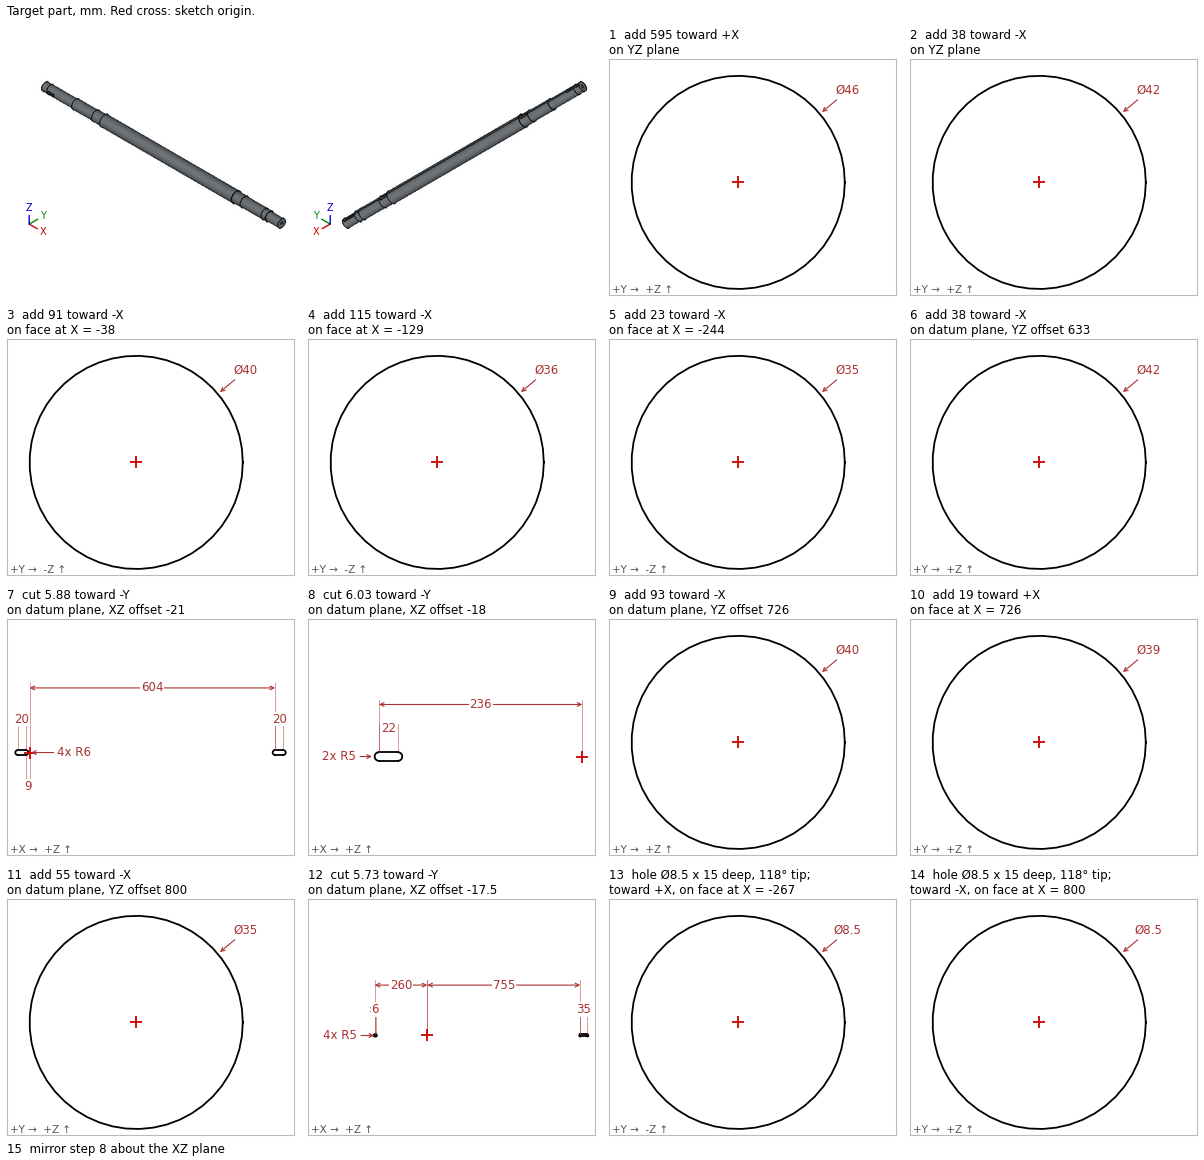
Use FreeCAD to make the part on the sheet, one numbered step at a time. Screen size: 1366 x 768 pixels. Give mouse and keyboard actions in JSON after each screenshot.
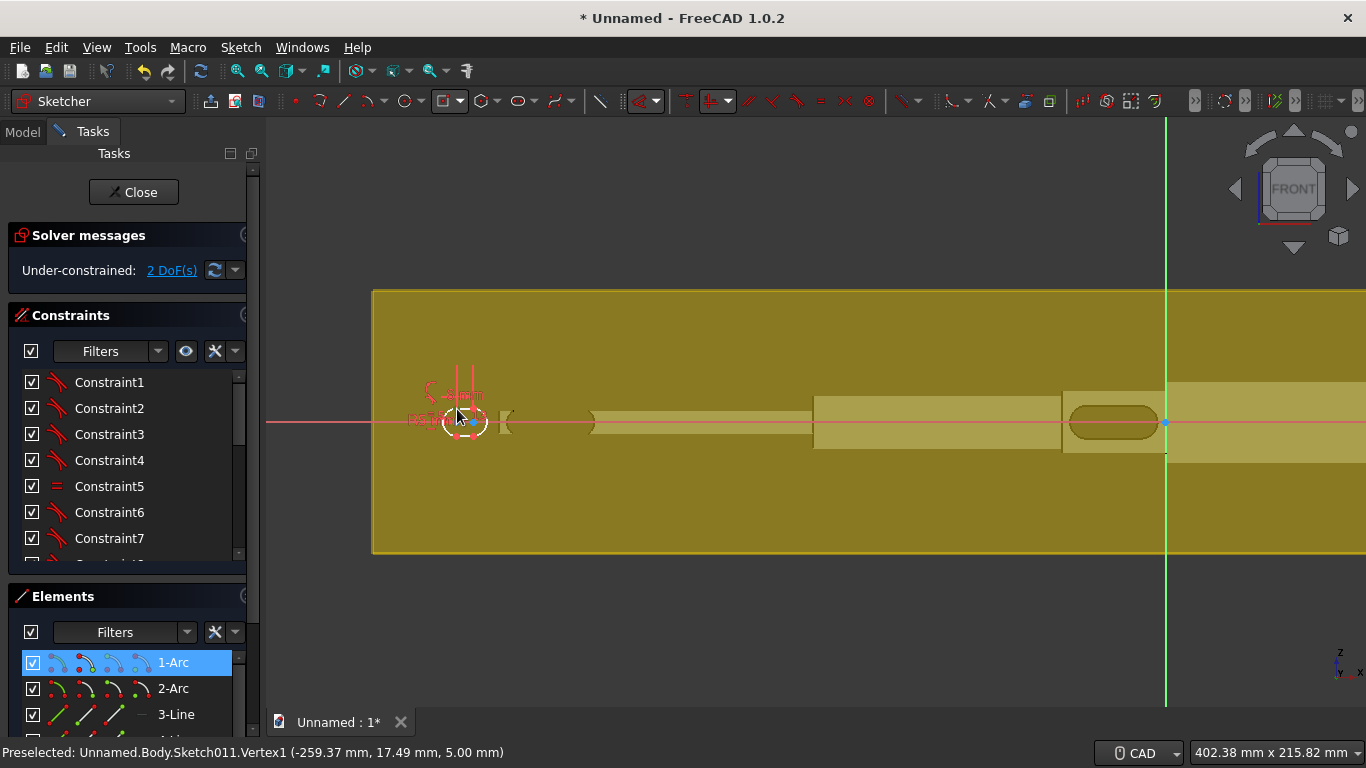
{"action": "key", "text": "l"}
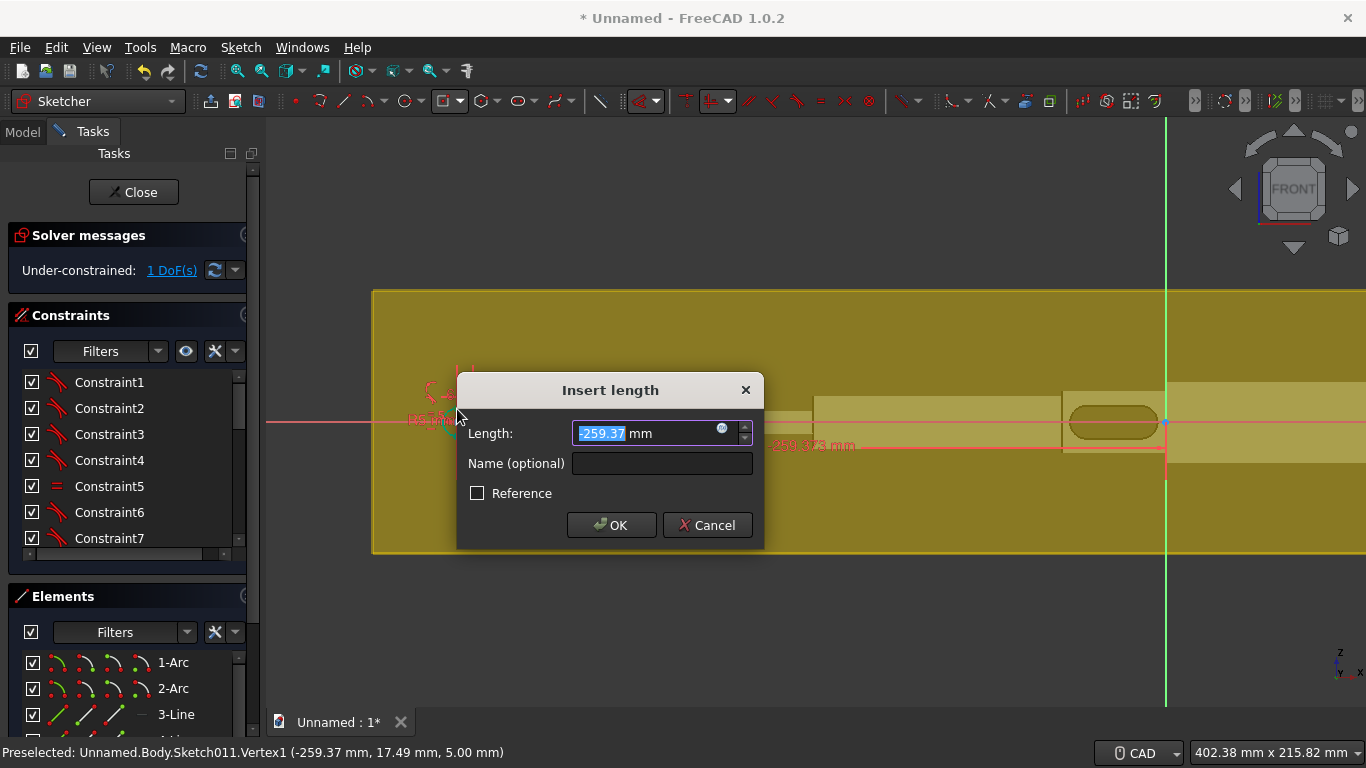
{"action": "type", "text": "-260"}
{"action": "key", "text": "Return"}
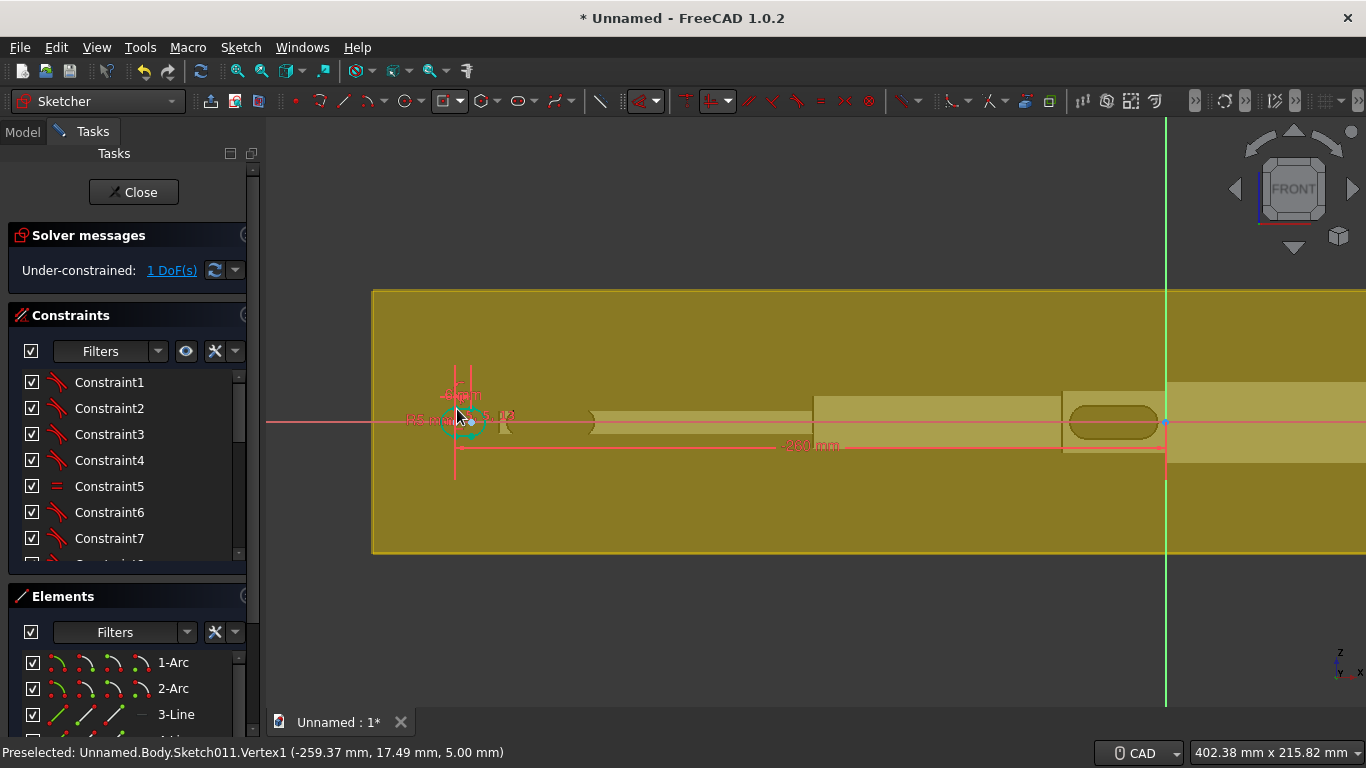
{"action": "scroll", "coordinate": [458, 409], "scroll_direction": "down", "scroll_amount": 8}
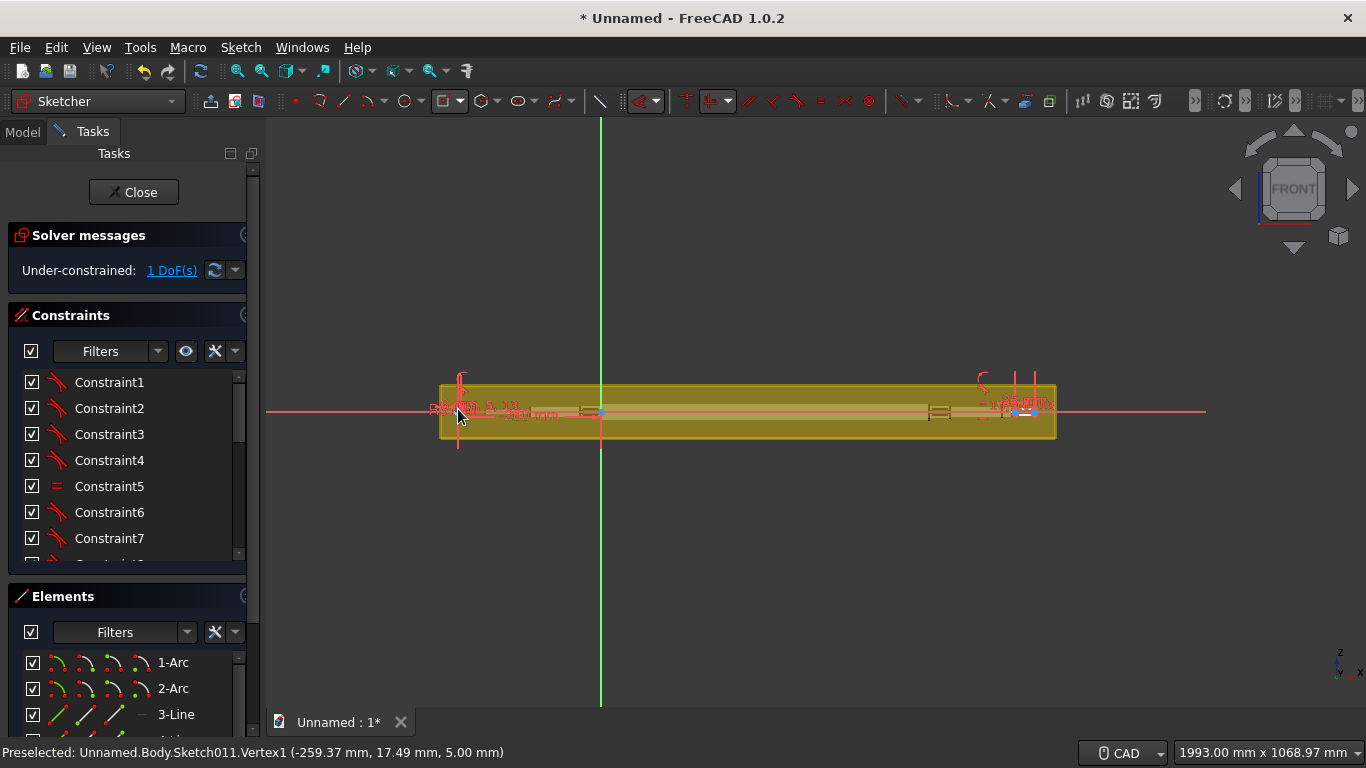
{"action": "scroll", "coordinate": [1015, 409], "scroll_direction": "up", "scroll_amount": 8}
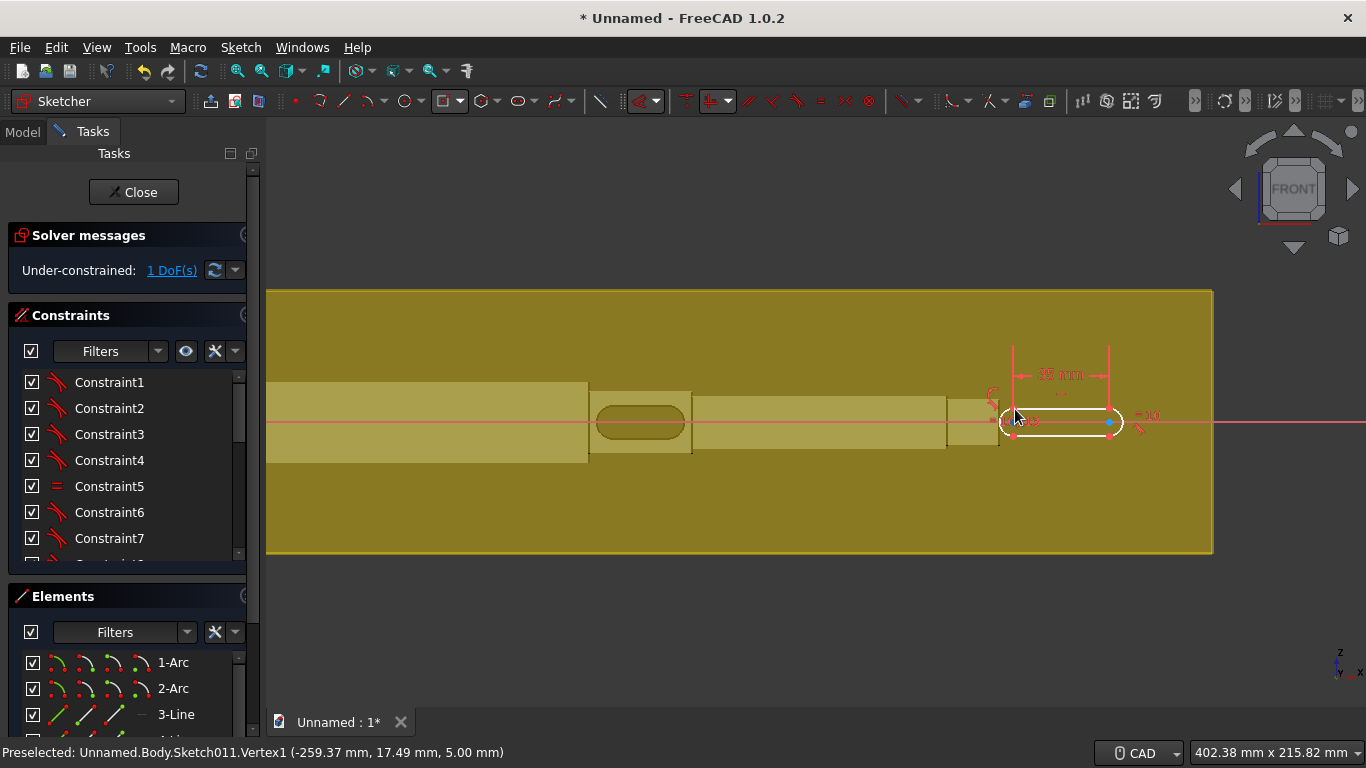
{"action": "left_click", "coordinate": [1013, 409]}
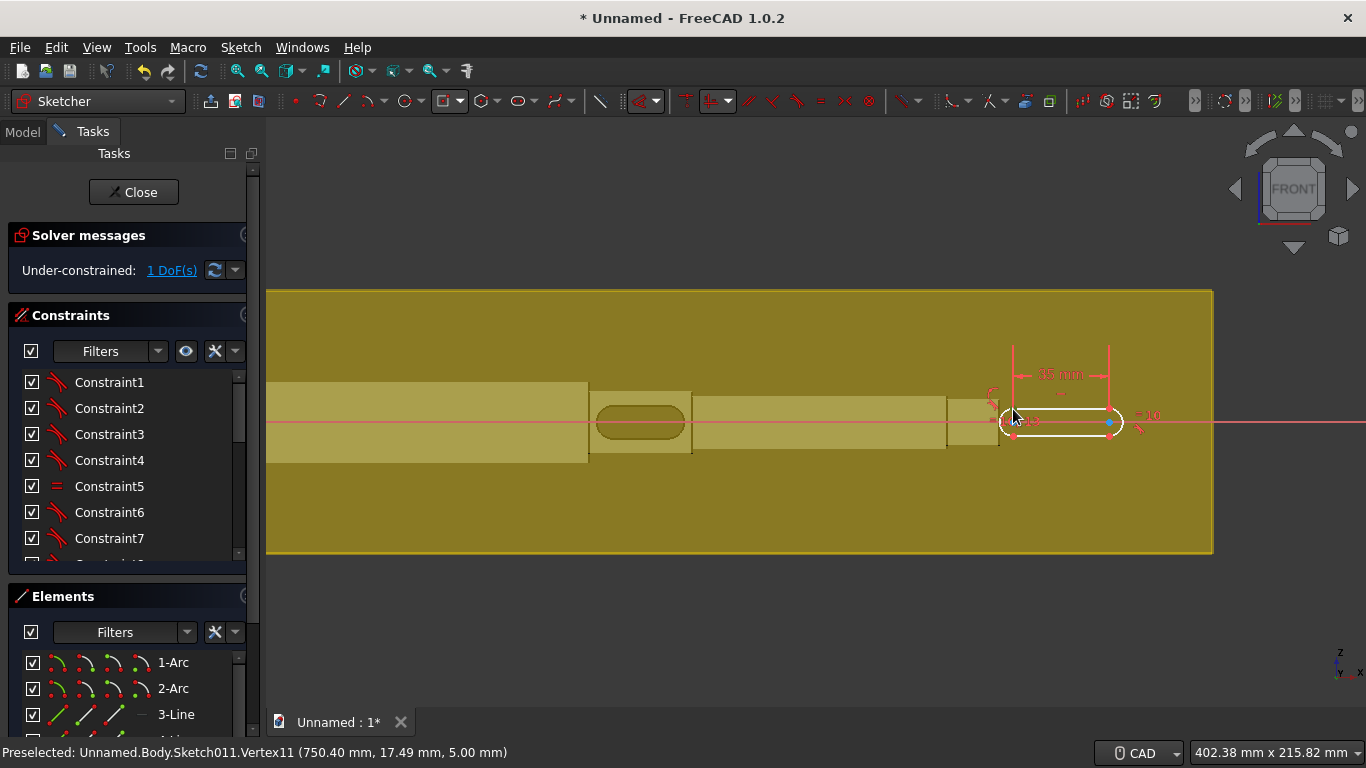
{"action": "key", "text": "l"}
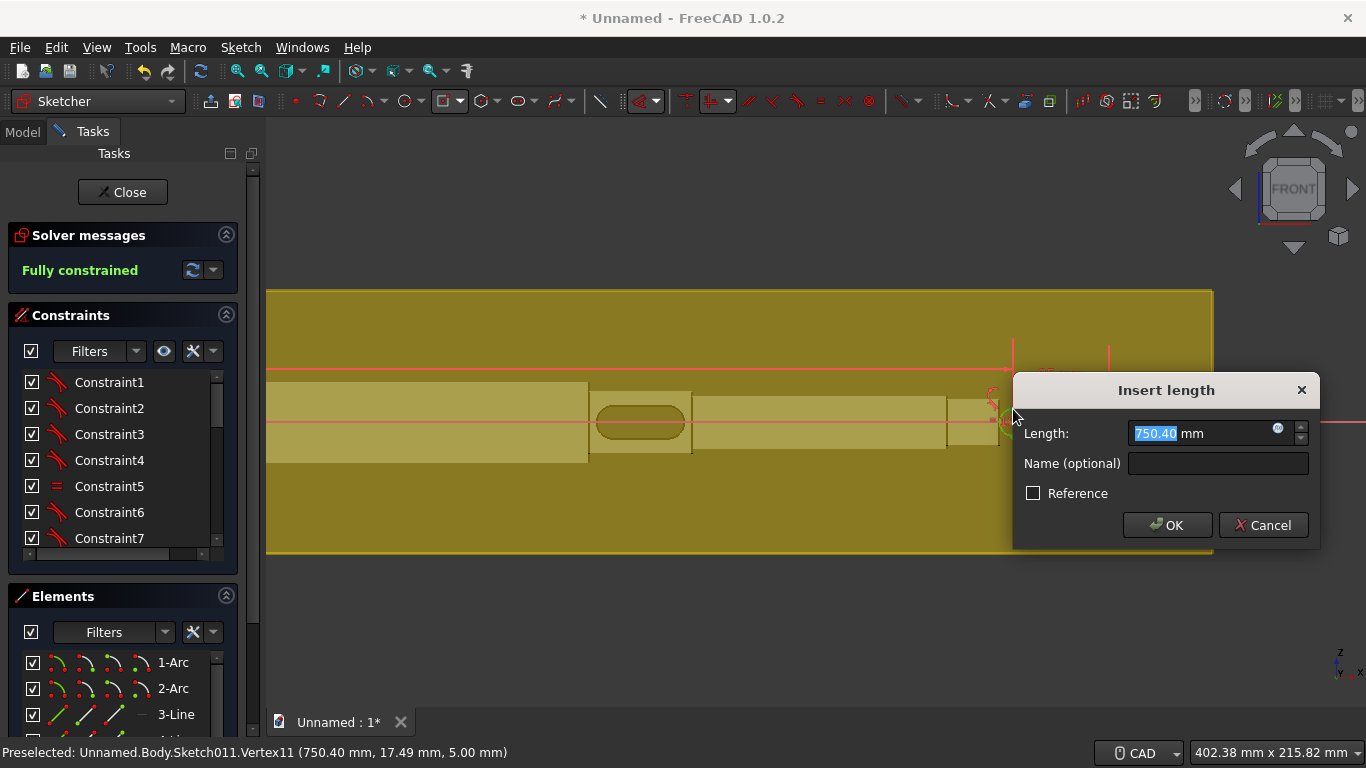
{"action": "type", "text": "755"}
{"action": "key", "text": "Return"}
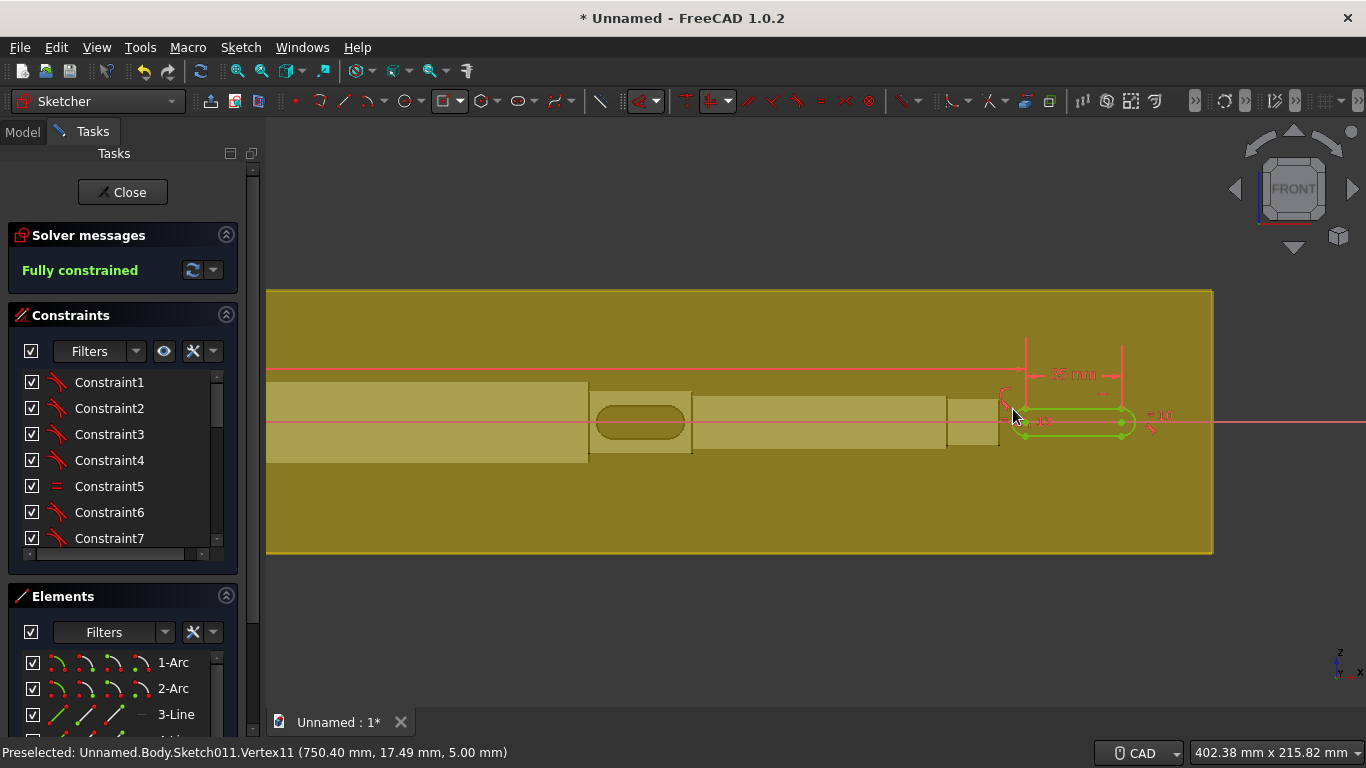
{"action": "left_click", "coordinate": [123, 192]}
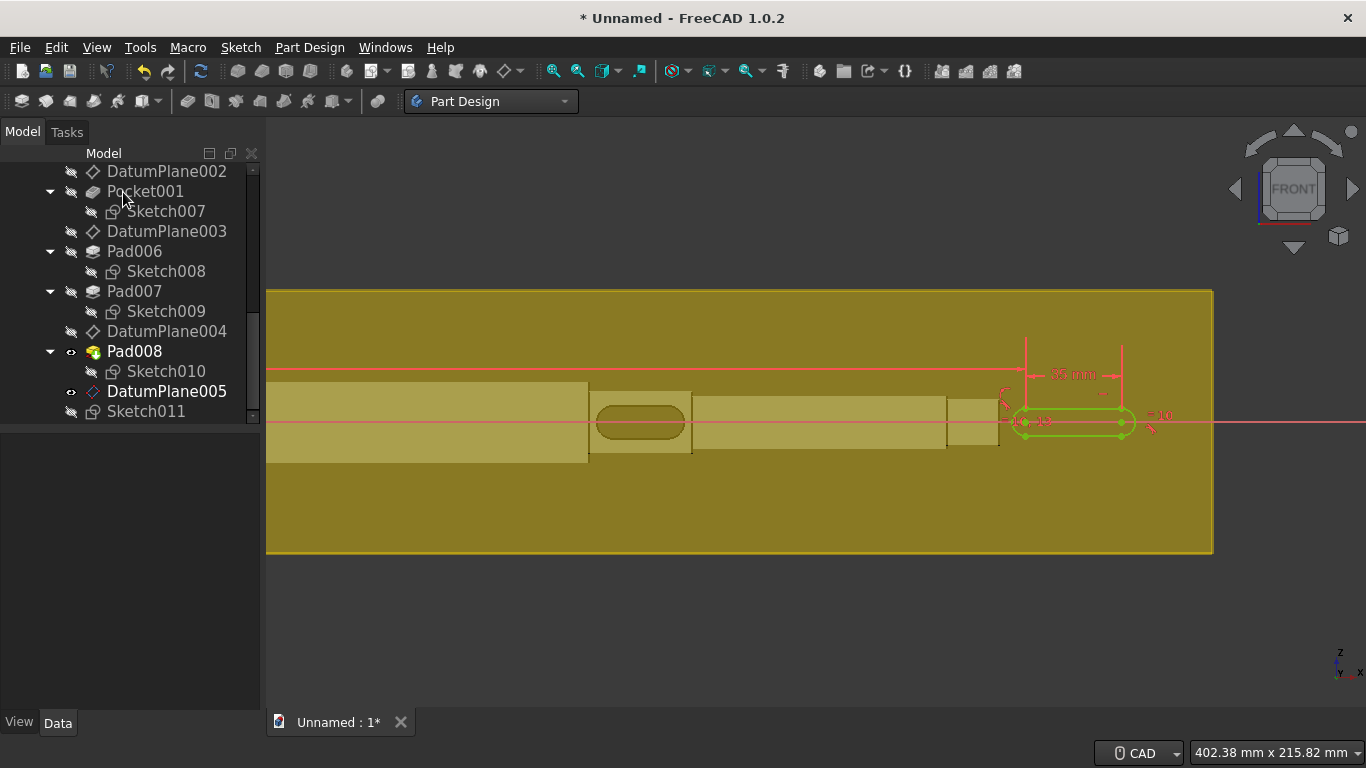
{"action": "left_click", "coordinate": [188, 102]}